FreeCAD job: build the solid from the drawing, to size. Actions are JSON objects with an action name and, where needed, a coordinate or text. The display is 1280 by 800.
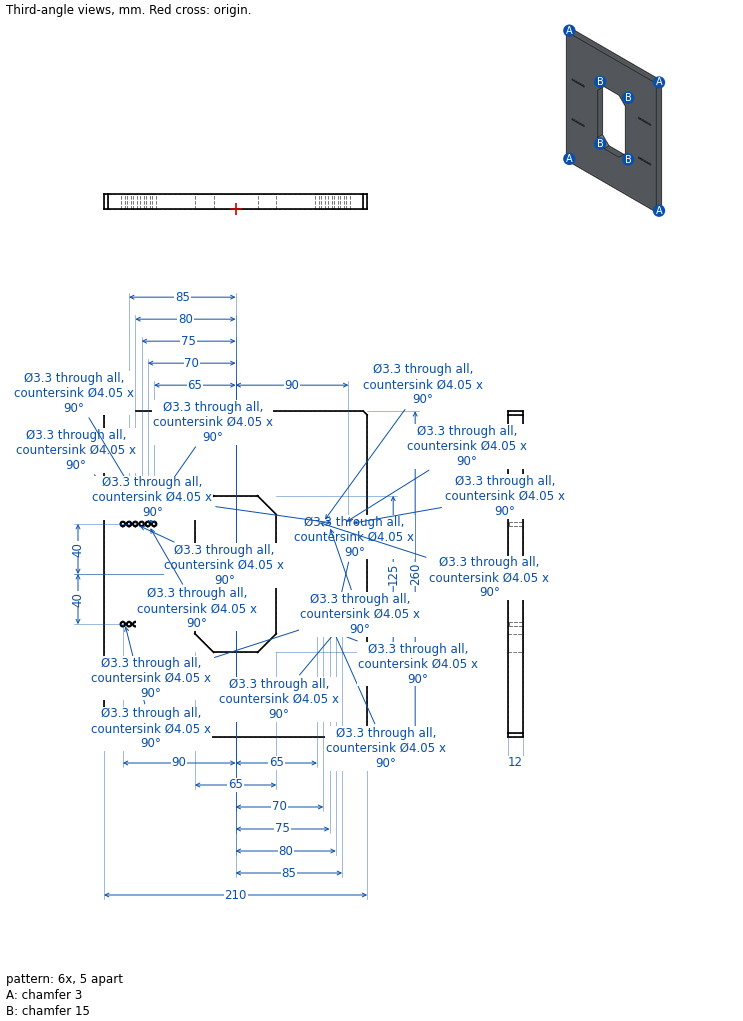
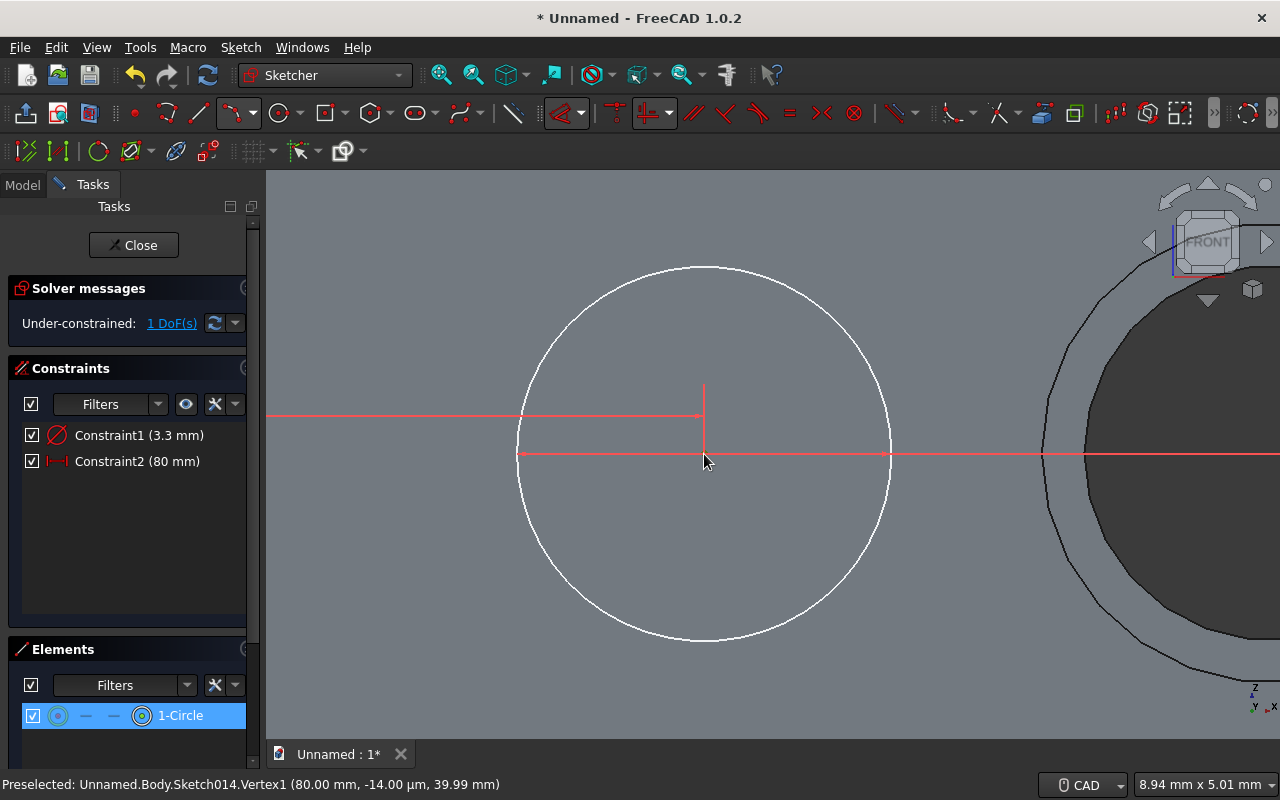
{"action": "left_click", "coordinate": [584, 114]}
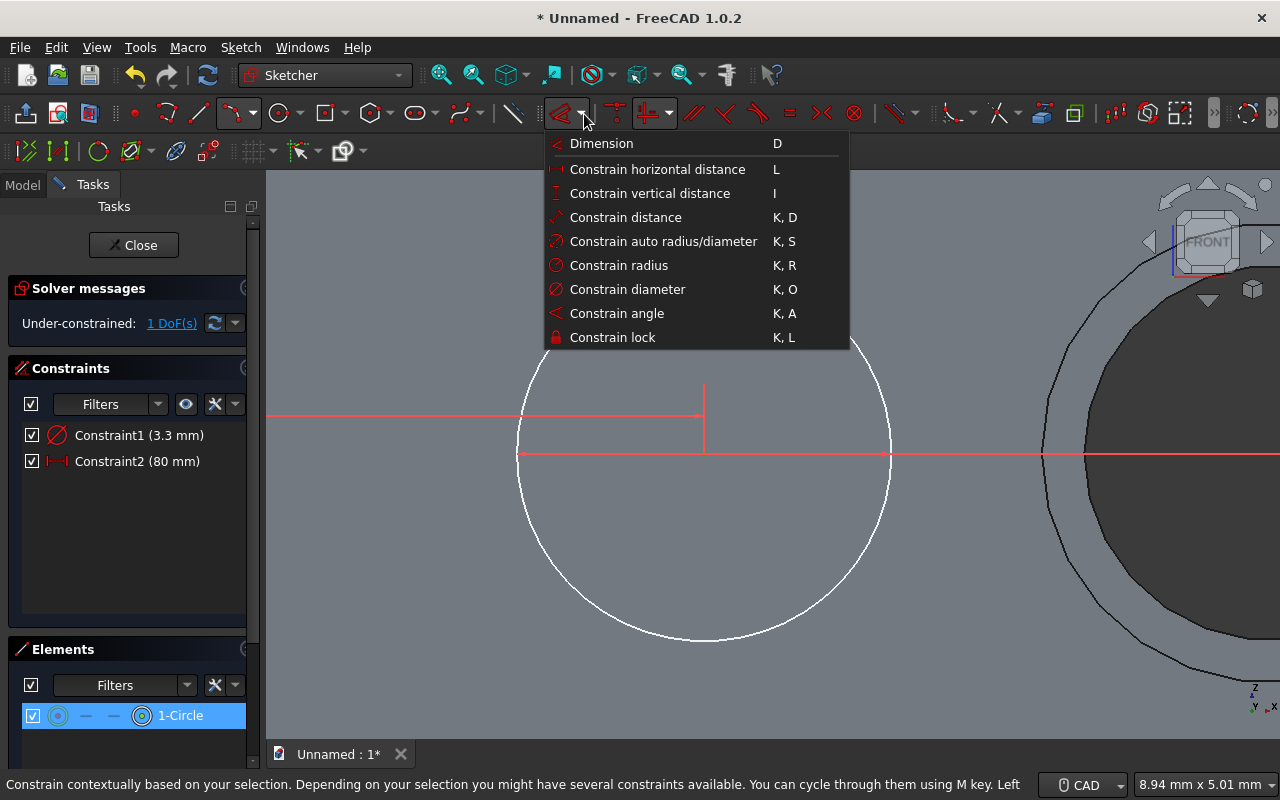
{"action": "left_click", "coordinate": [697, 193]}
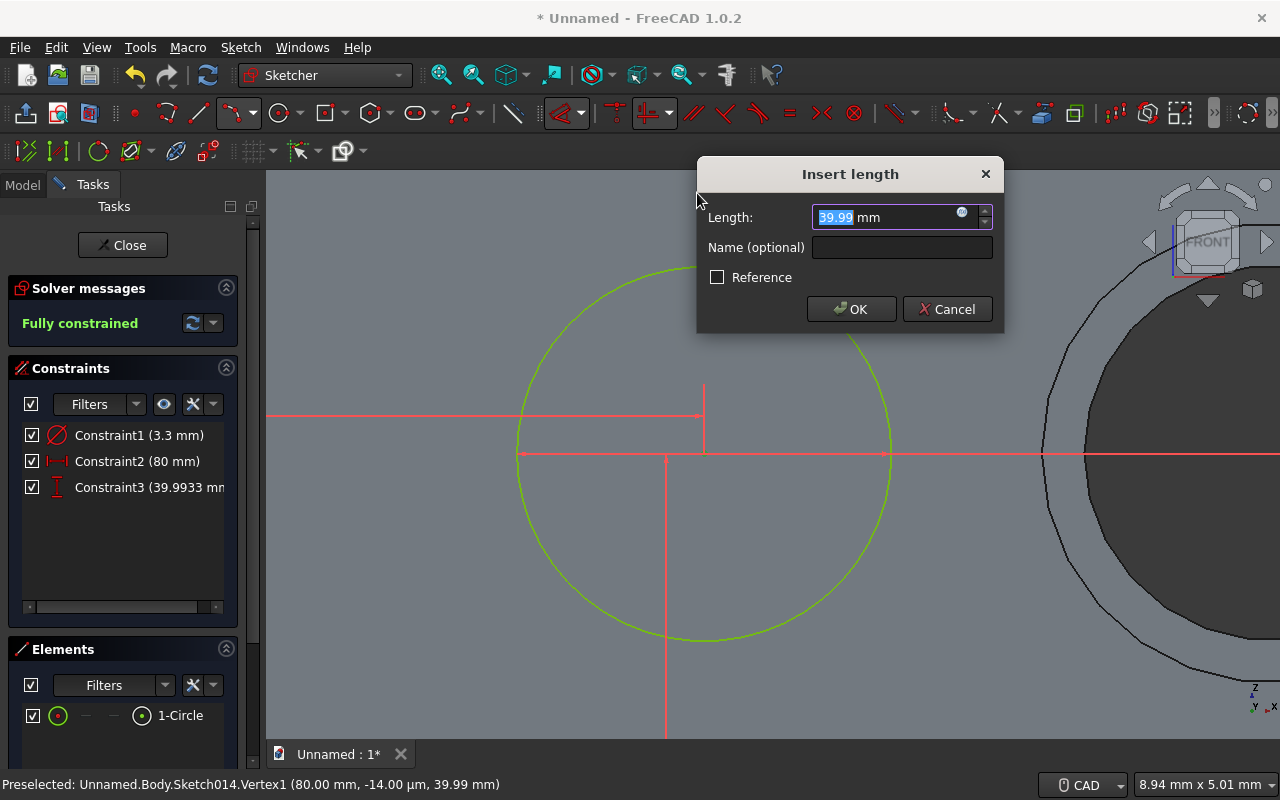
{"action": "type", "text": "40"}
{"action": "key", "text": "Return"}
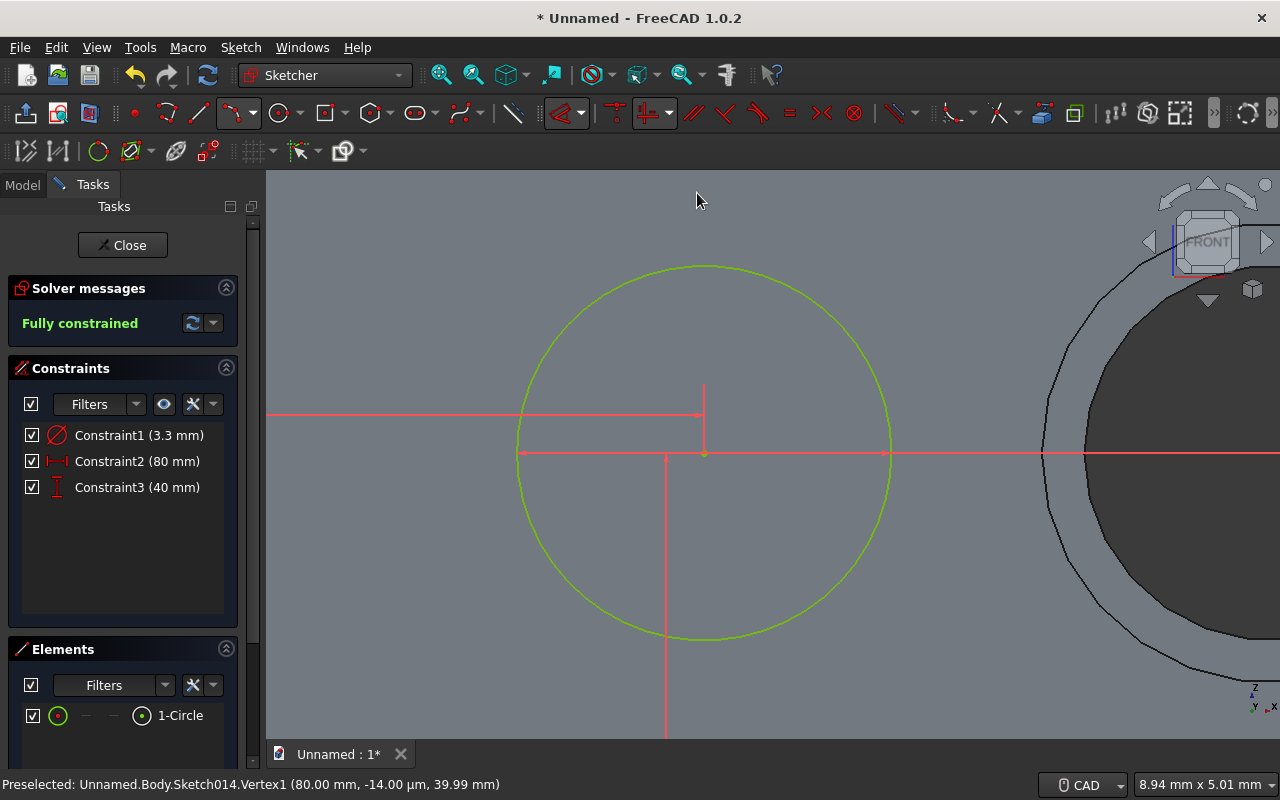
{"action": "left_click", "coordinate": [123, 245]}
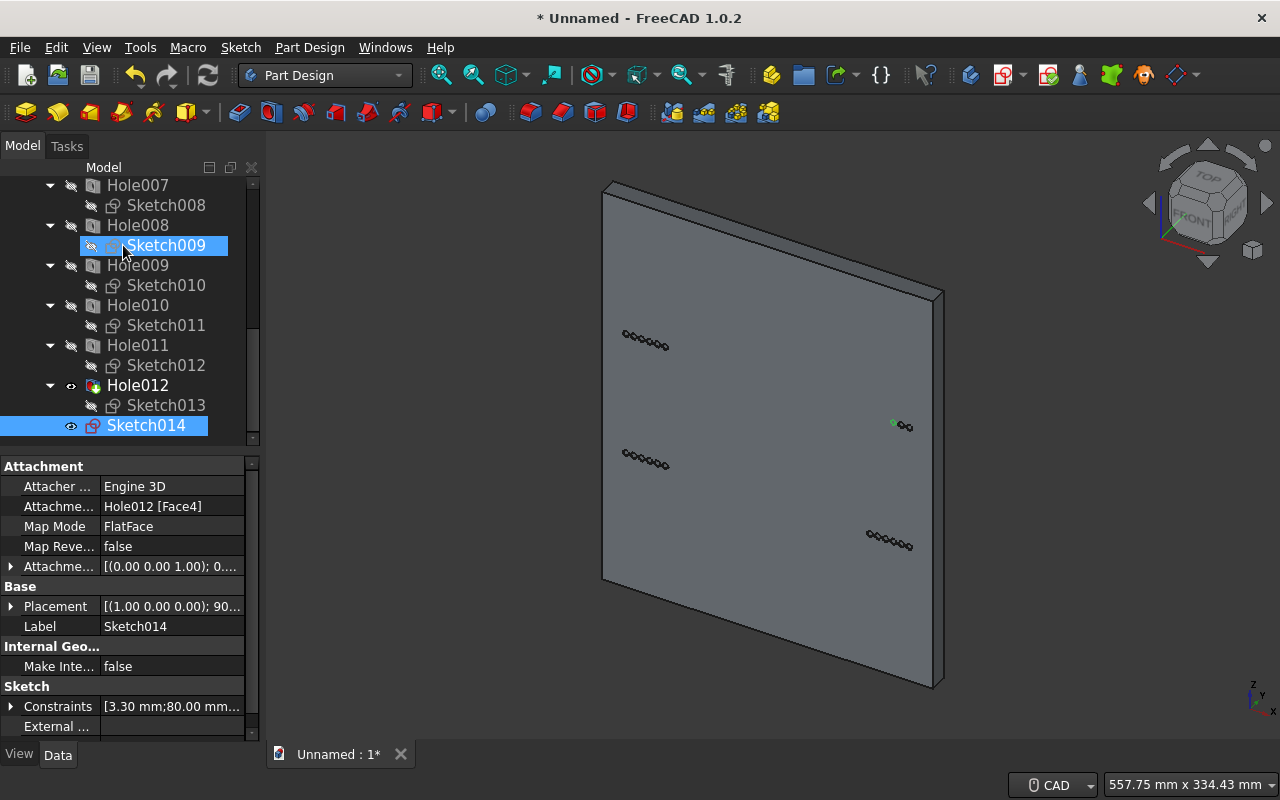
{"action": "left_click", "coordinate": [272, 112]}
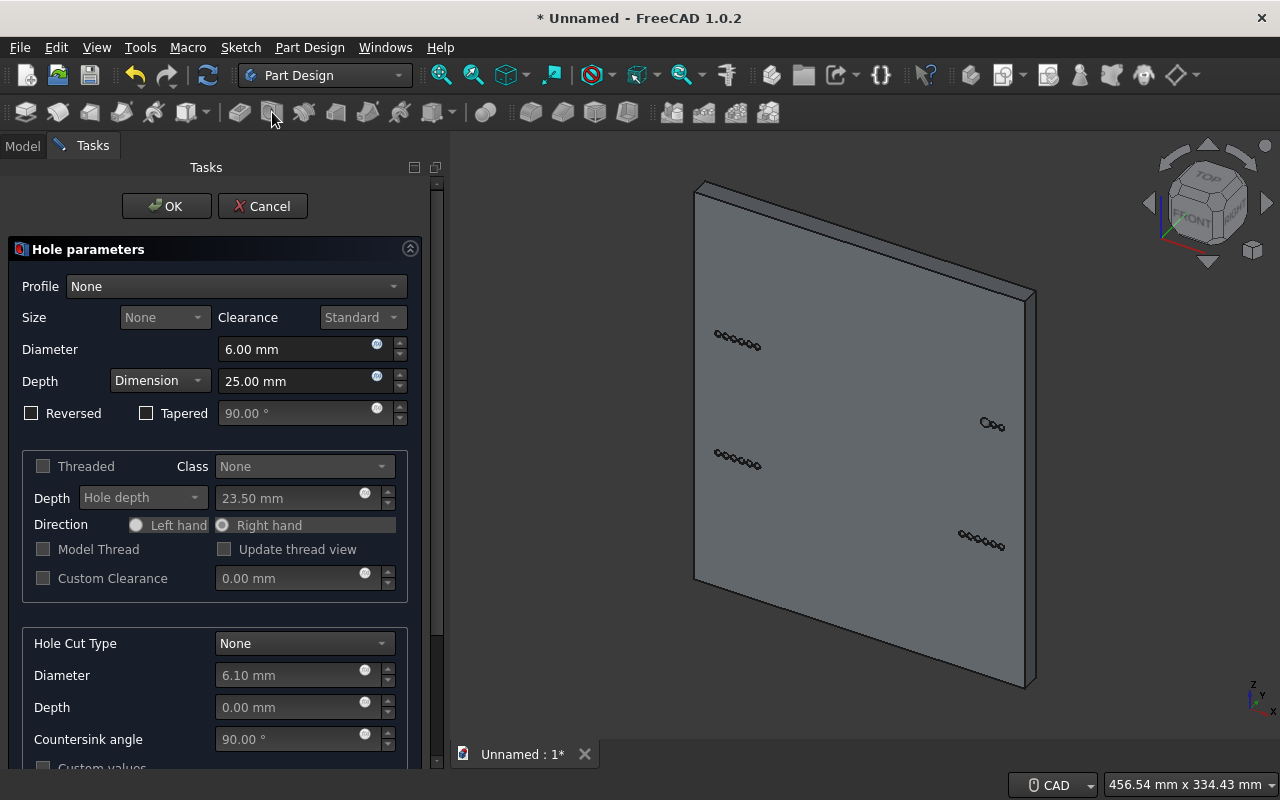
{"action": "triple_click", "coordinate": [305, 349]}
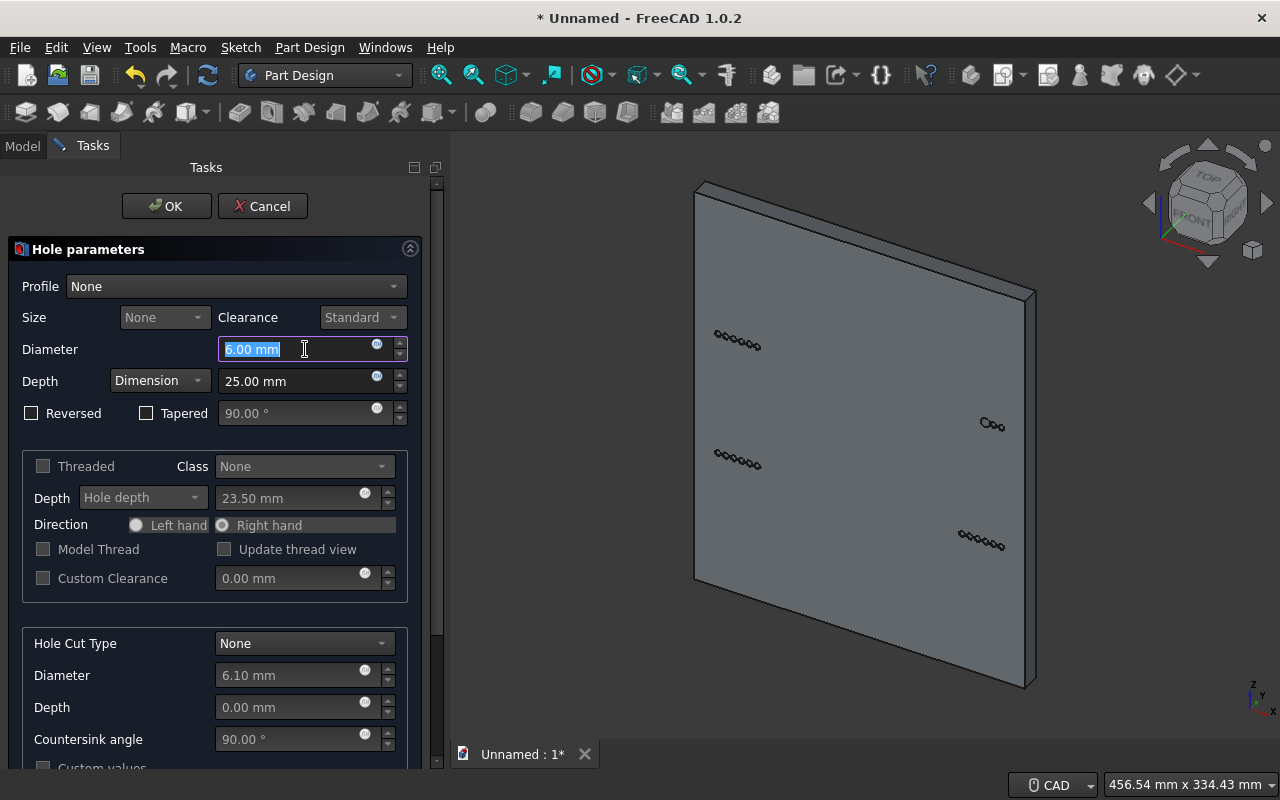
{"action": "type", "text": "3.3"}
{"action": "key", "text": "Tab"}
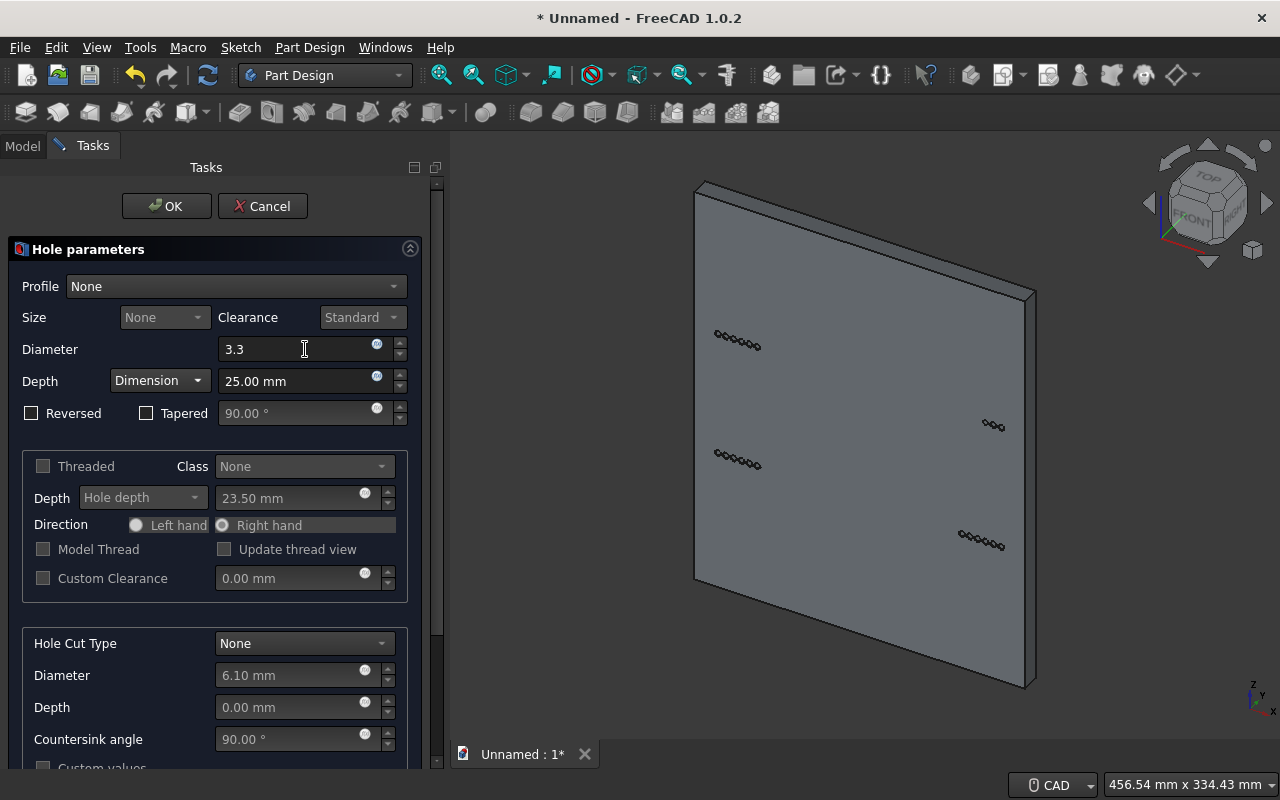
{"action": "left_click", "coordinate": [161, 380]}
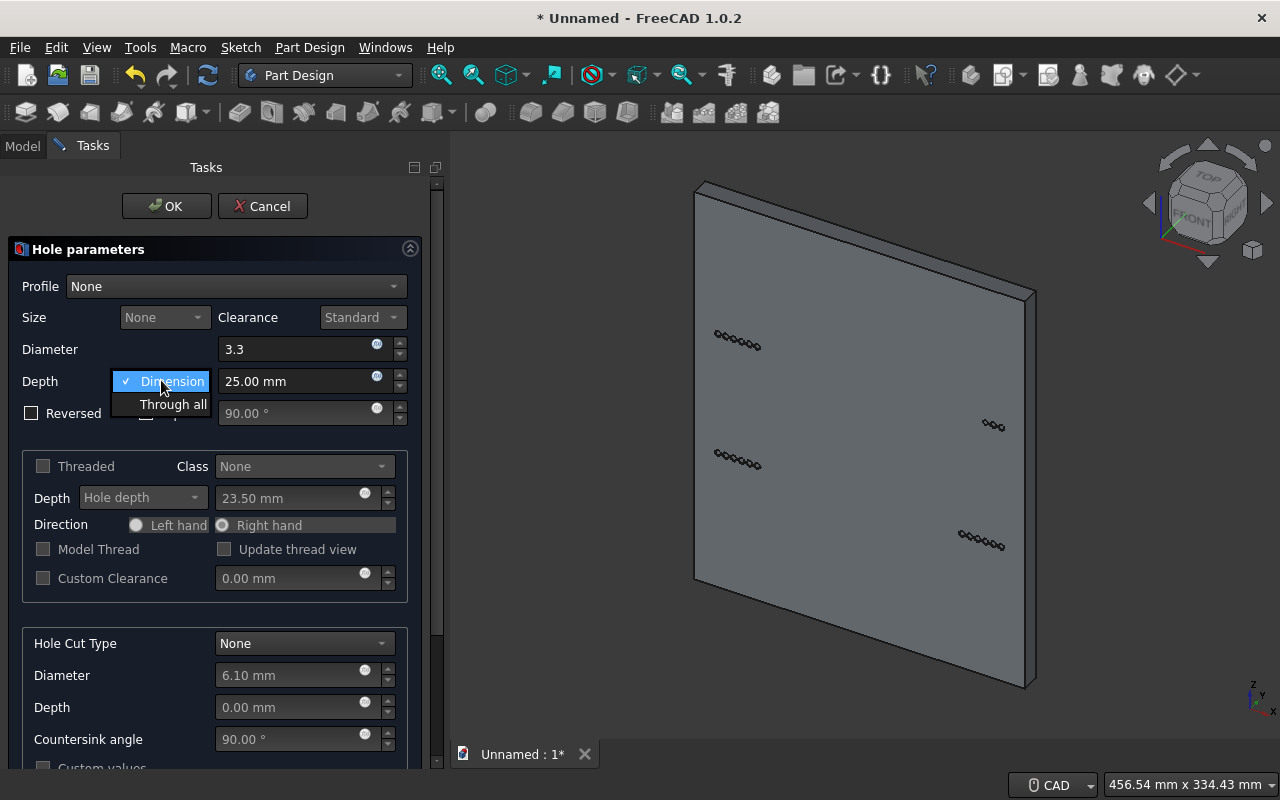
{"action": "left_click", "coordinate": [160, 404]}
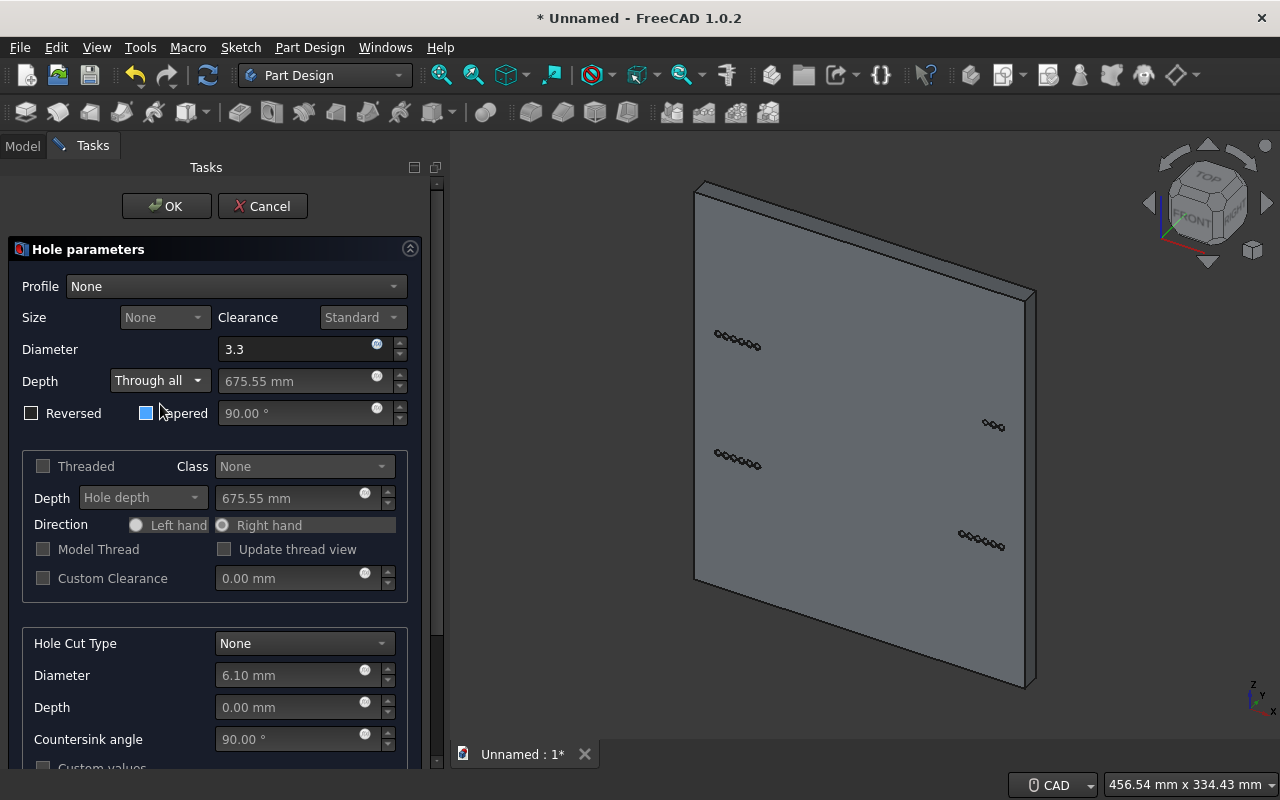
{"action": "left_click", "coordinate": [306, 644]}